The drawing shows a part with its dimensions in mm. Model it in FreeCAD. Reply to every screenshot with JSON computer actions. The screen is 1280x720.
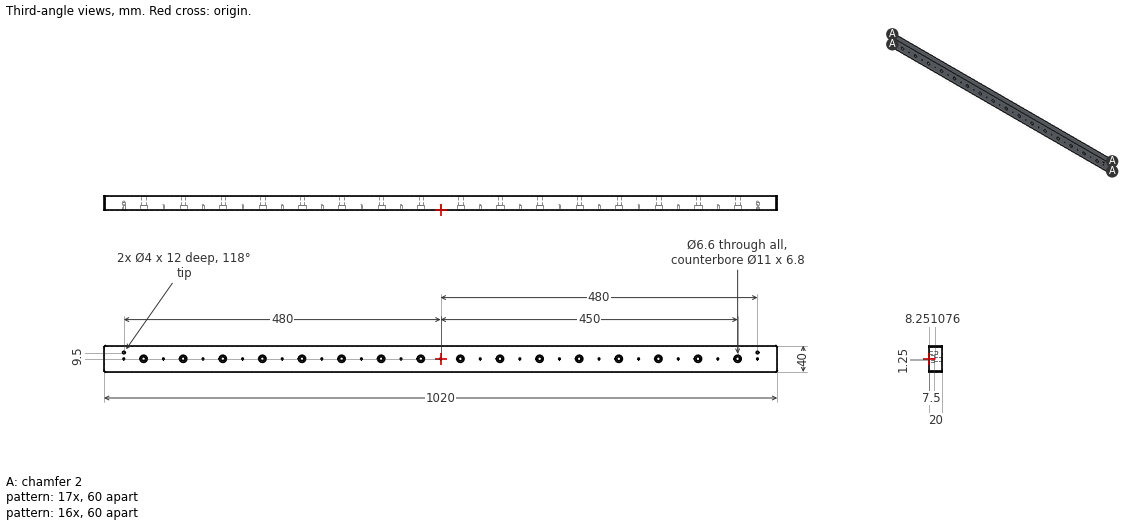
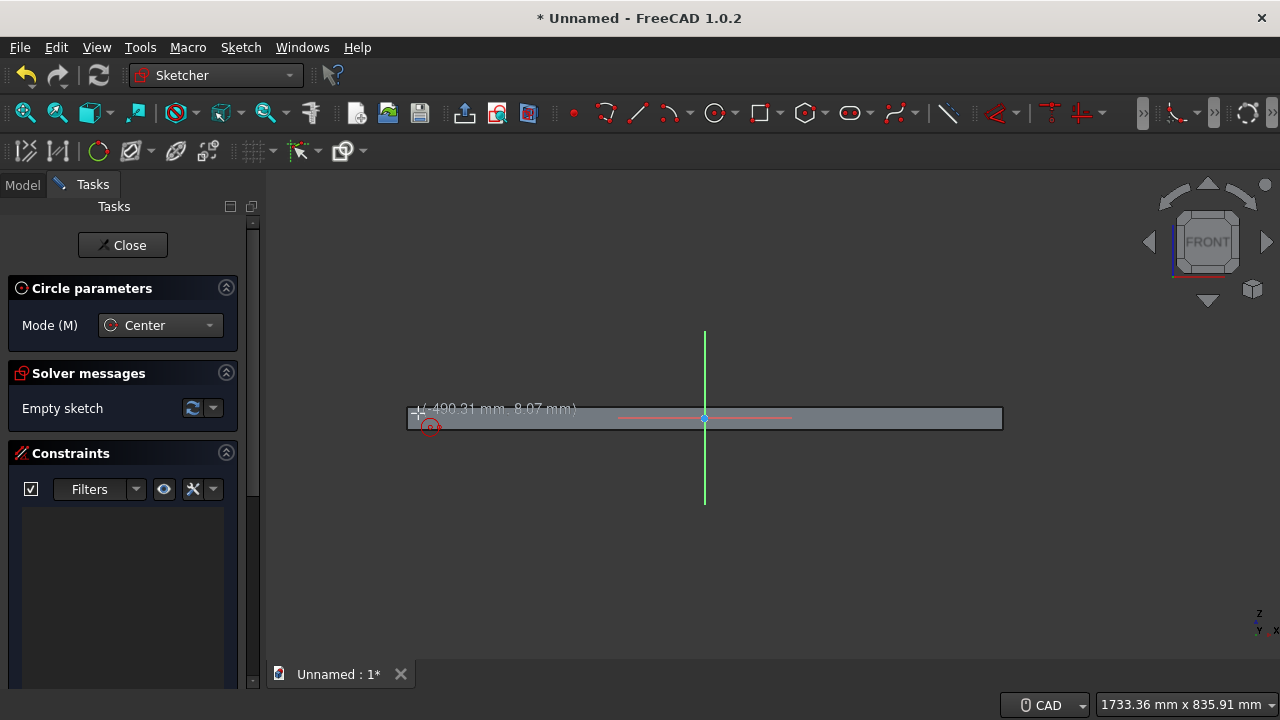
{"action": "scroll", "coordinate": [424, 413], "scroll_direction": "up", "scroll_amount": 6}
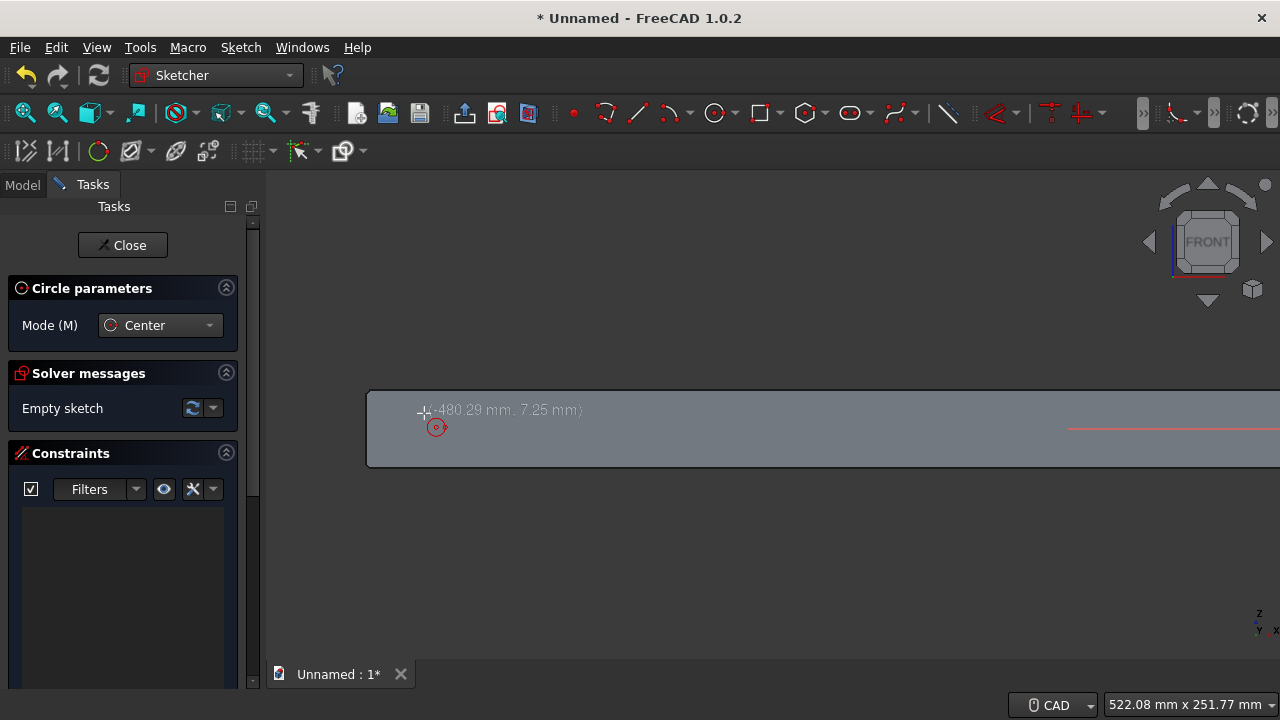
{"action": "left_click", "coordinate": [424, 411]}
{"action": "mouse_move", "coordinate": [427, 408]}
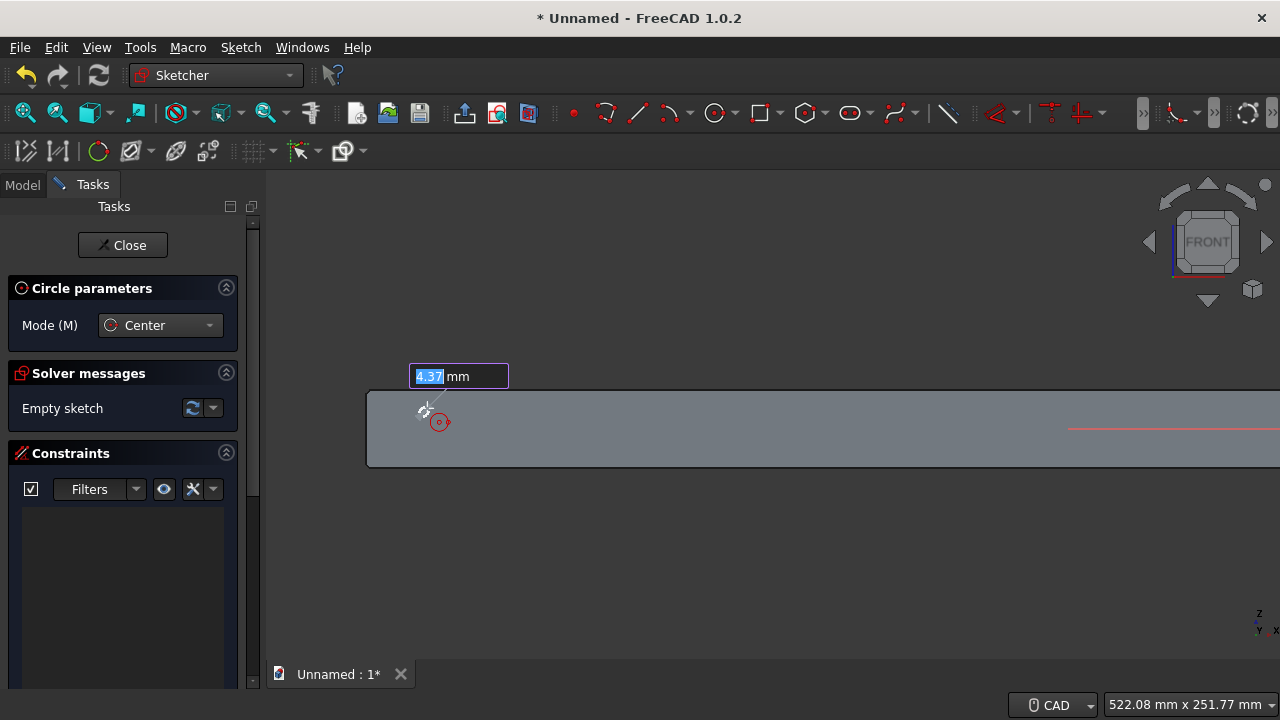
{"action": "type", "text": "4"}
{"action": "key", "text": "Return"}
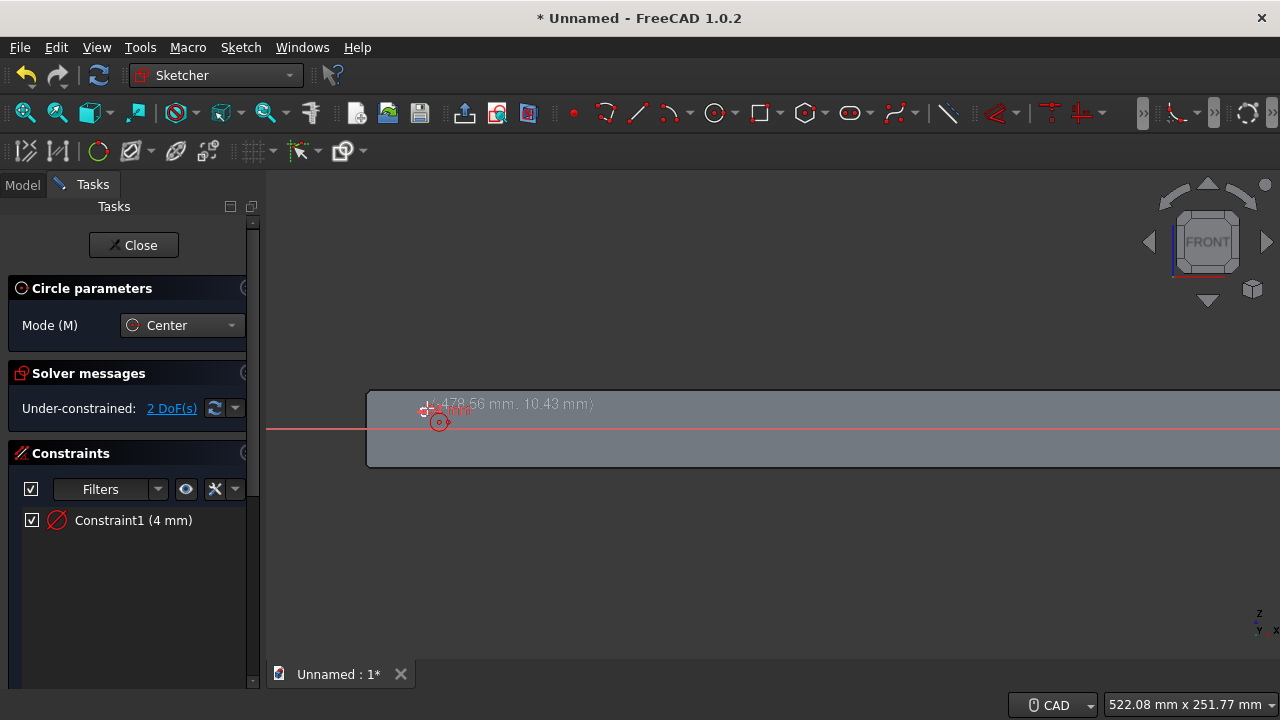
{"action": "scroll", "coordinate": [423, 413], "scroll_direction": "down", "scroll_amount": 6}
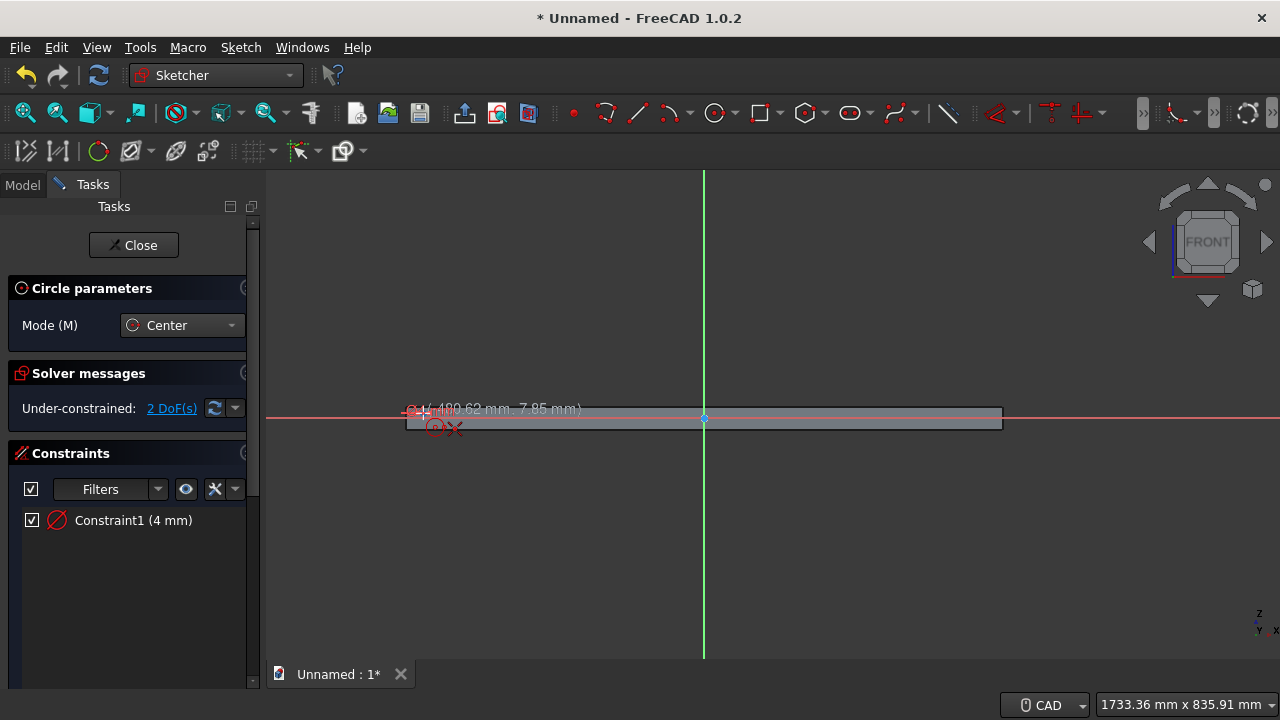
{"action": "scroll", "coordinate": [985, 413], "scroll_direction": "up", "scroll_amount": 15}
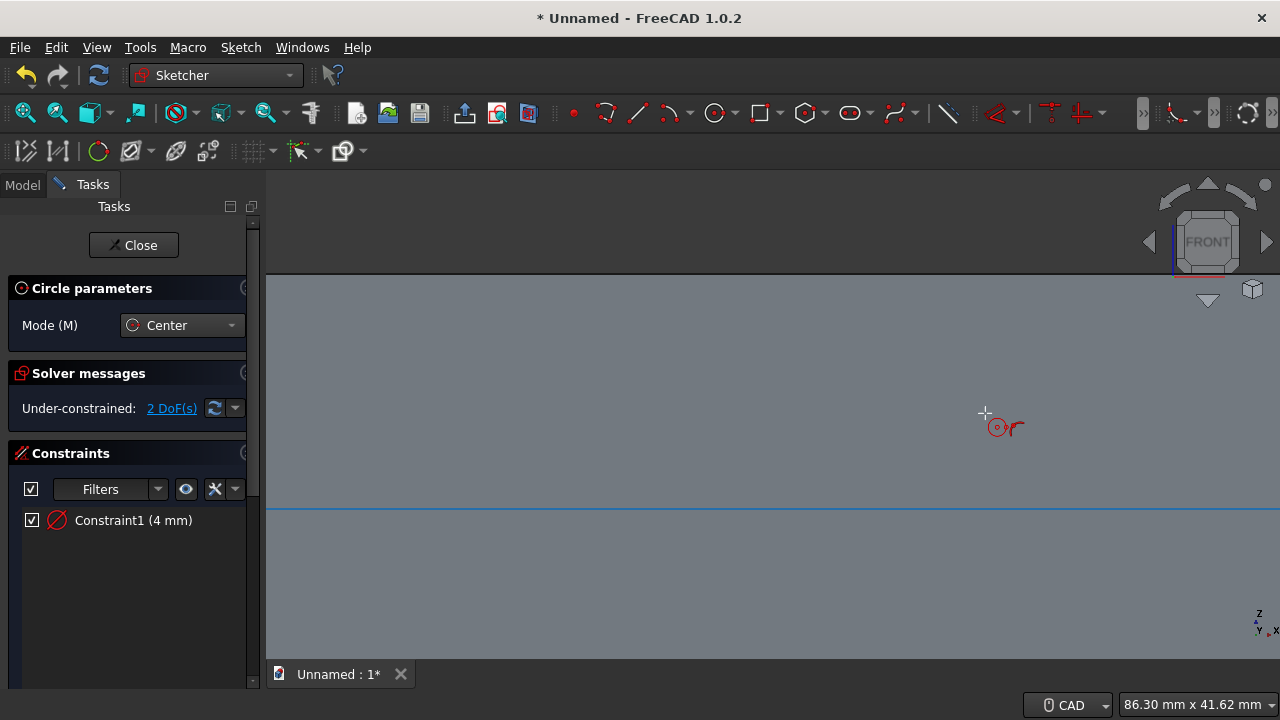
{"action": "scroll", "coordinate": [986, 413], "scroll_direction": "down", "scroll_amount": 15}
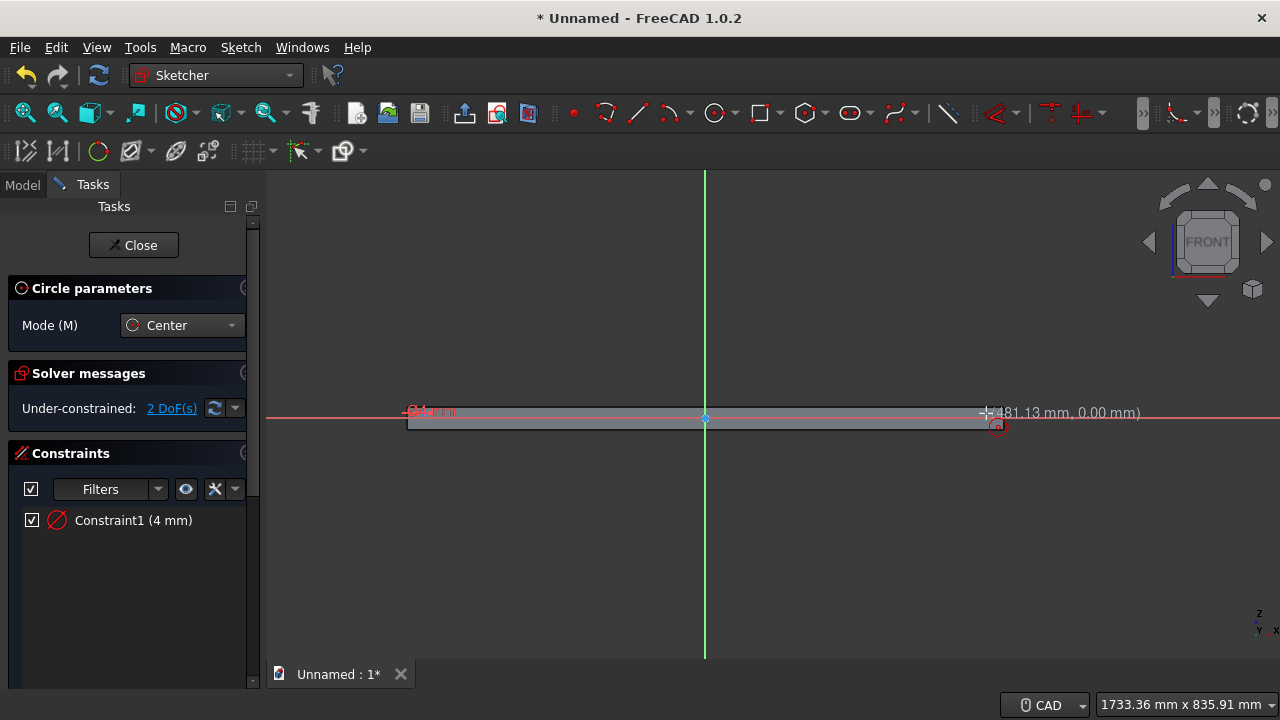
{"action": "scroll", "coordinate": [986, 413], "scroll_direction": "up", "scroll_amount": 6}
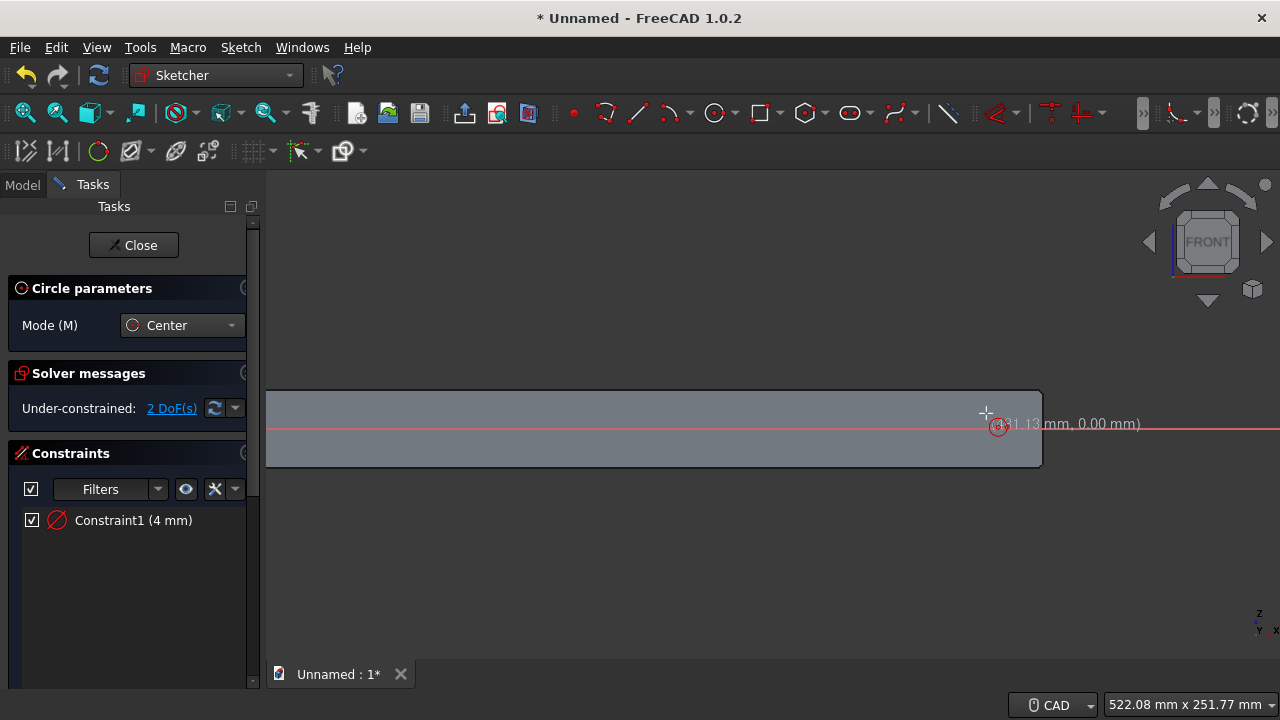
{"action": "left_click", "coordinate": [984, 411]}
{"action": "mouse_move", "coordinate": [987, 408]}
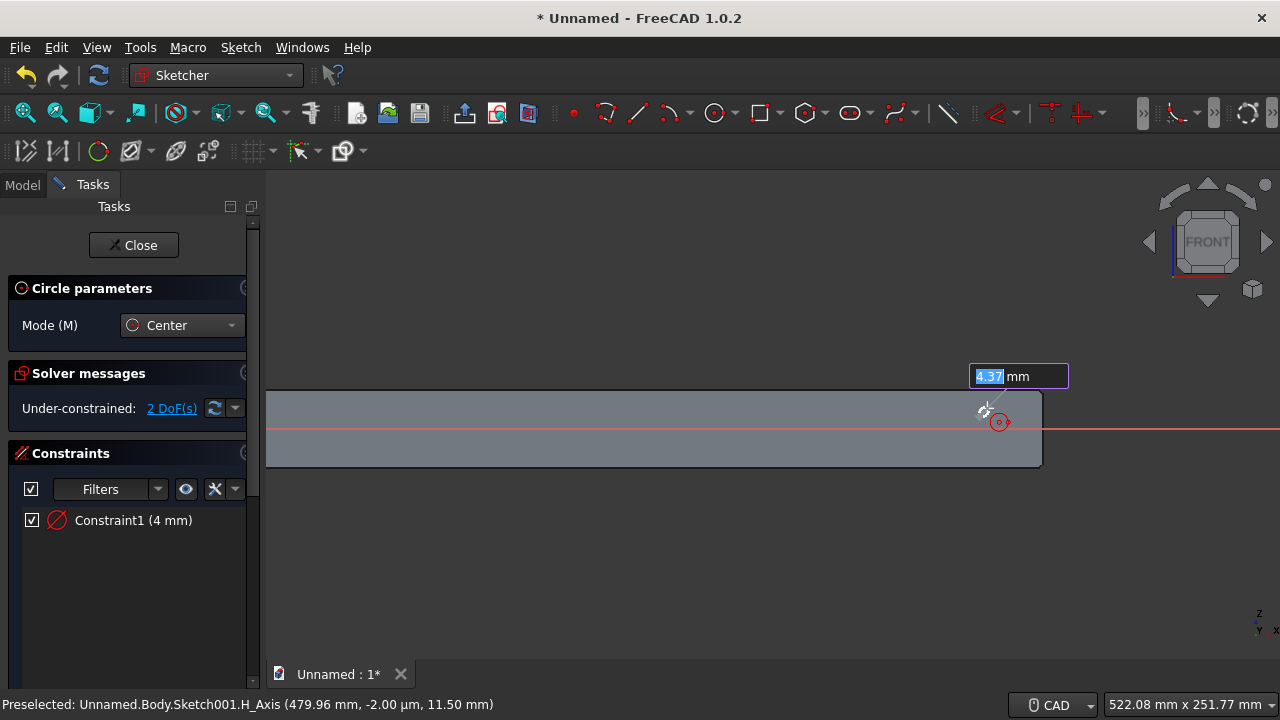
{"action": "type", "text": "4"}
{"action": "key", "text": "Return"}
{"action": "key", "text": "Escape"}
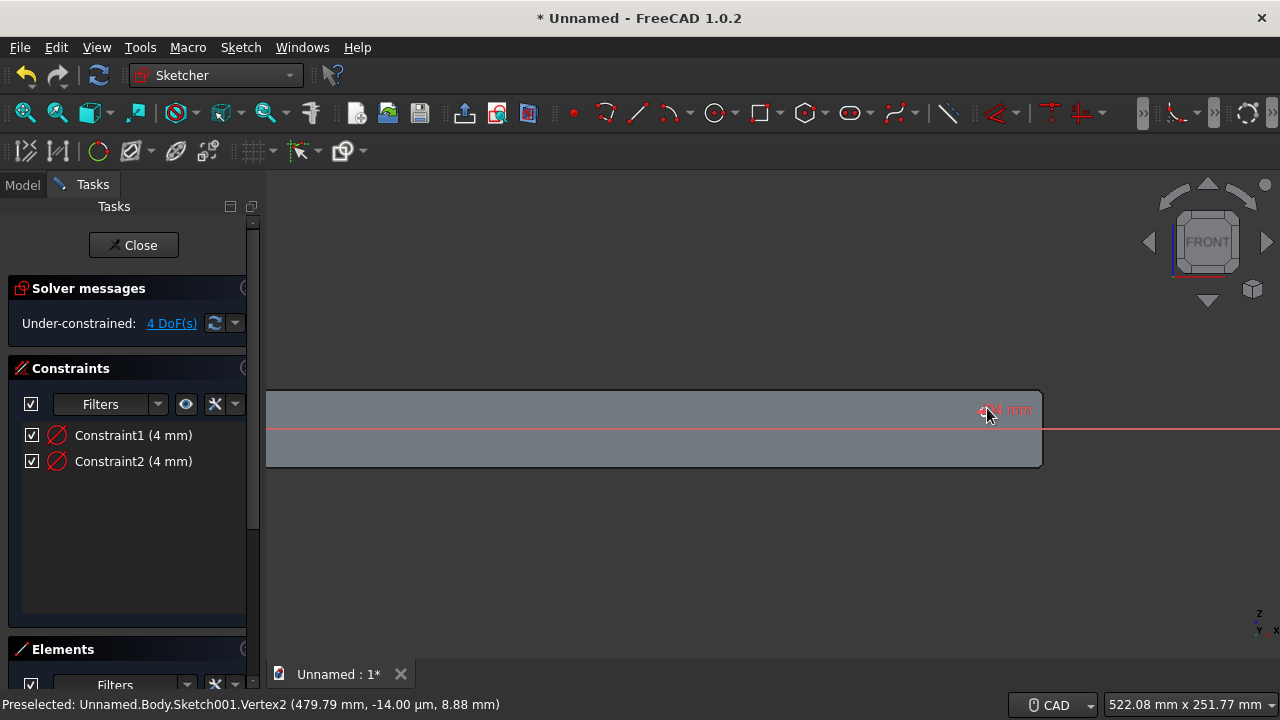
{"action": "scroll", "coordinate": [986, 413], "scroll_direction": "down", "scroll_amount": 6}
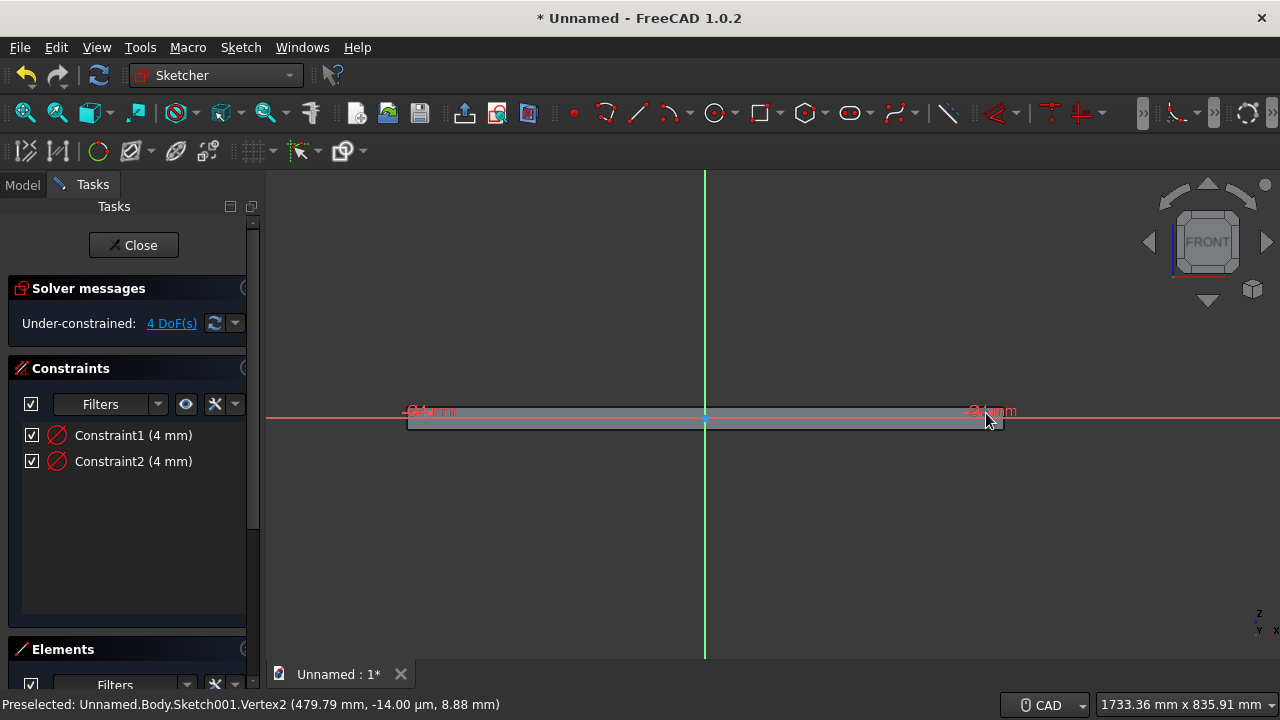
{"action": "left_click", "coordinate": [424, 413]}